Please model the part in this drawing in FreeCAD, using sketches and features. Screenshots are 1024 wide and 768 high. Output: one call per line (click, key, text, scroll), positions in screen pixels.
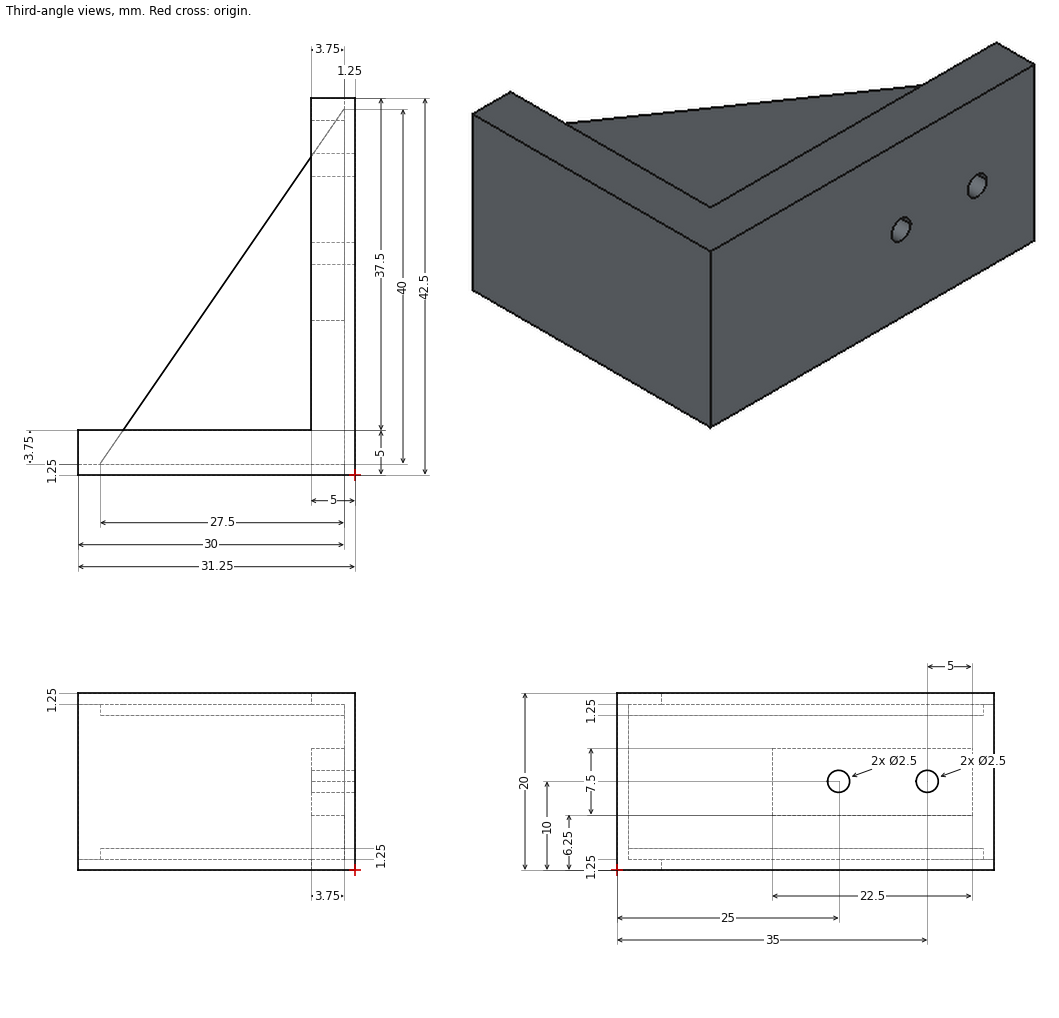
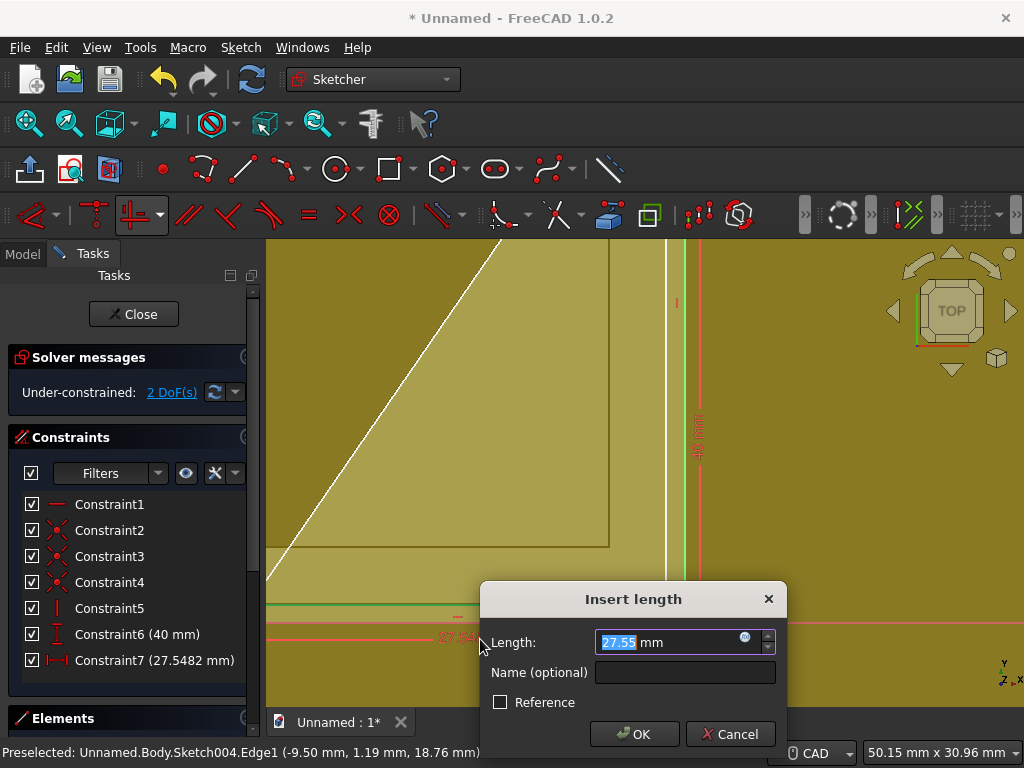
text(27.5)
key(Return)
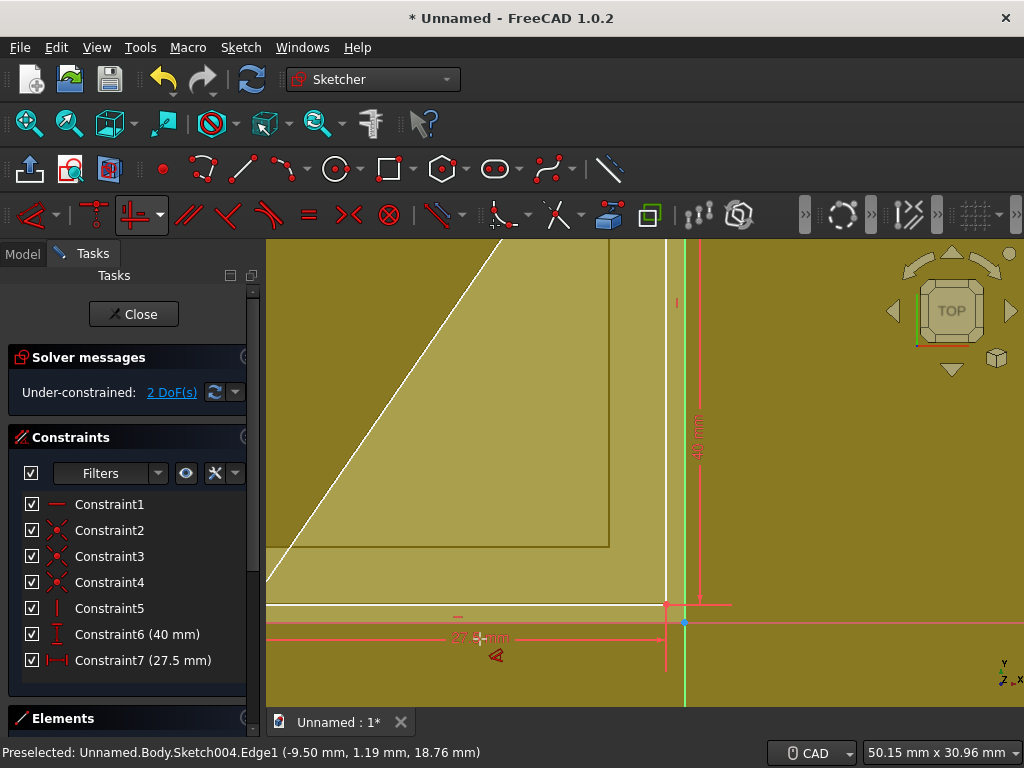
scroll(666, 605, up, 4)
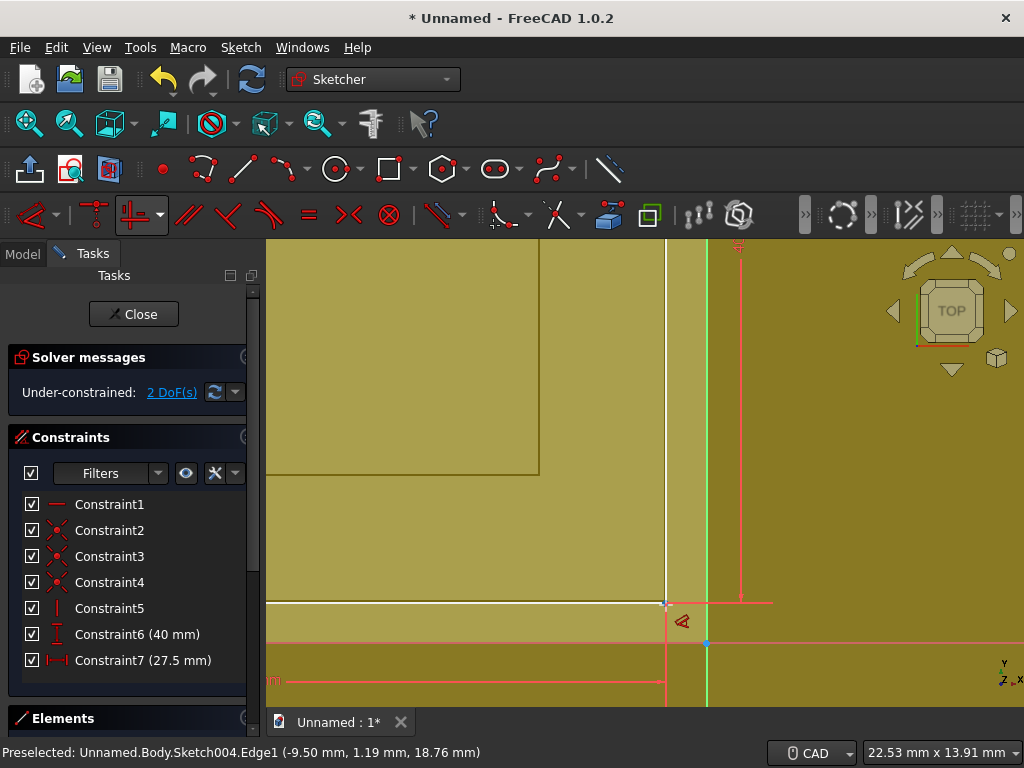
click(666, 603)
click(686, 677)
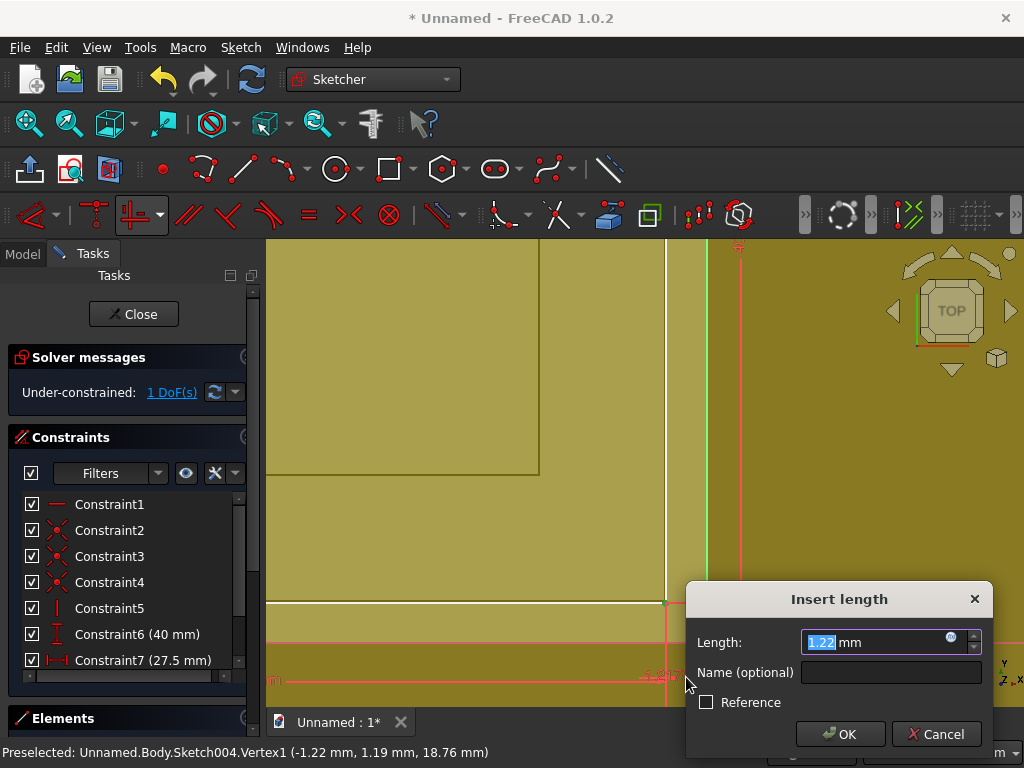
text(1.25)
key(Return)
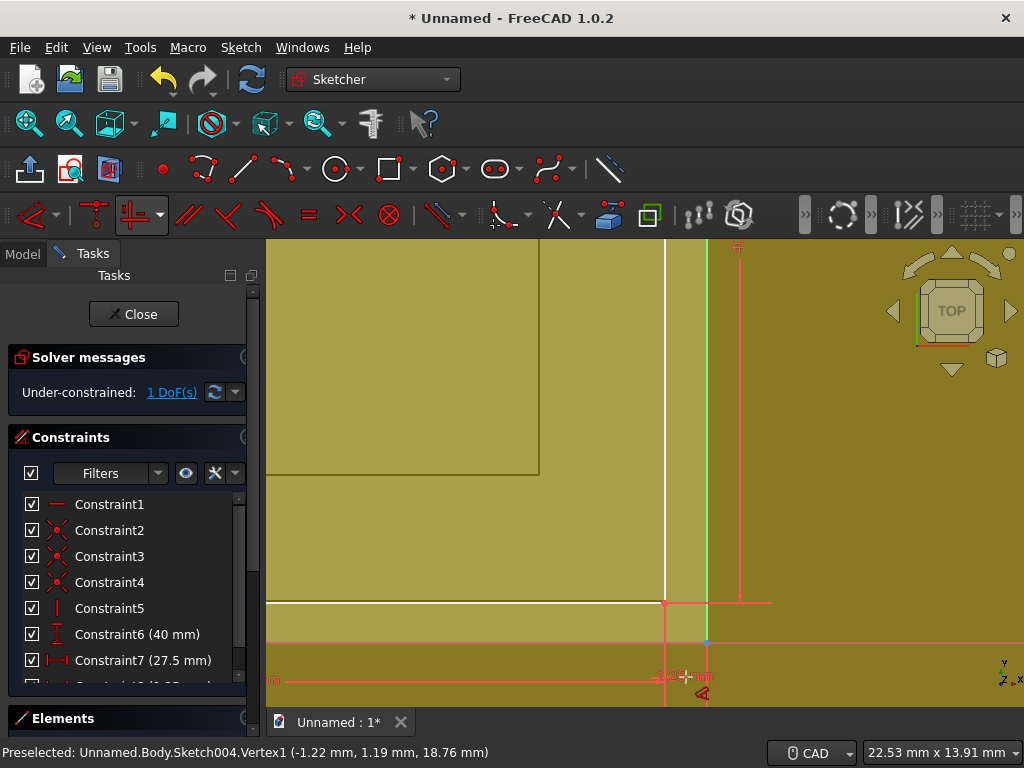
click(665, 603)
click(741, 623)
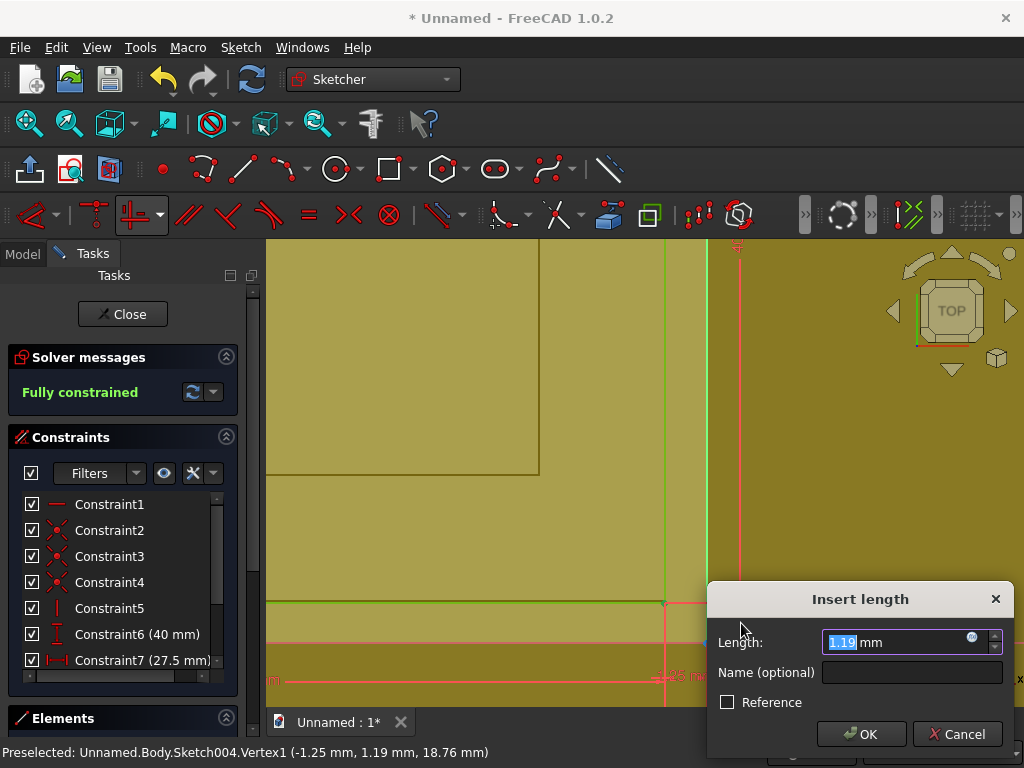
text(1.25)
key(Return)
key(Escape)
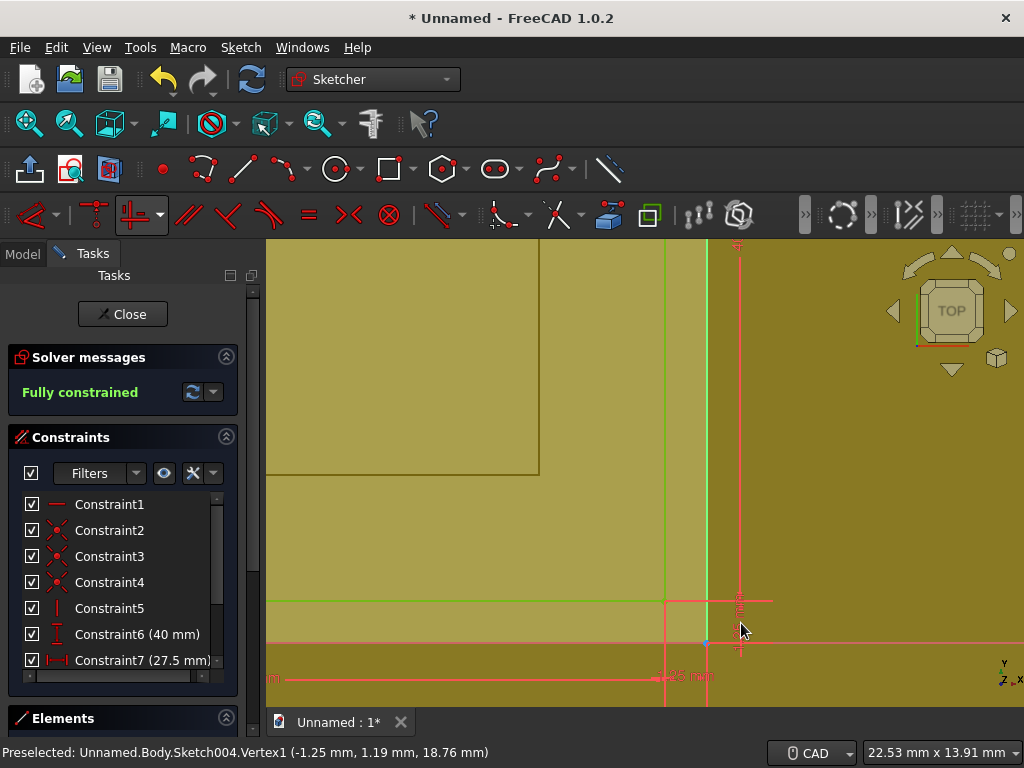
click(123, 314)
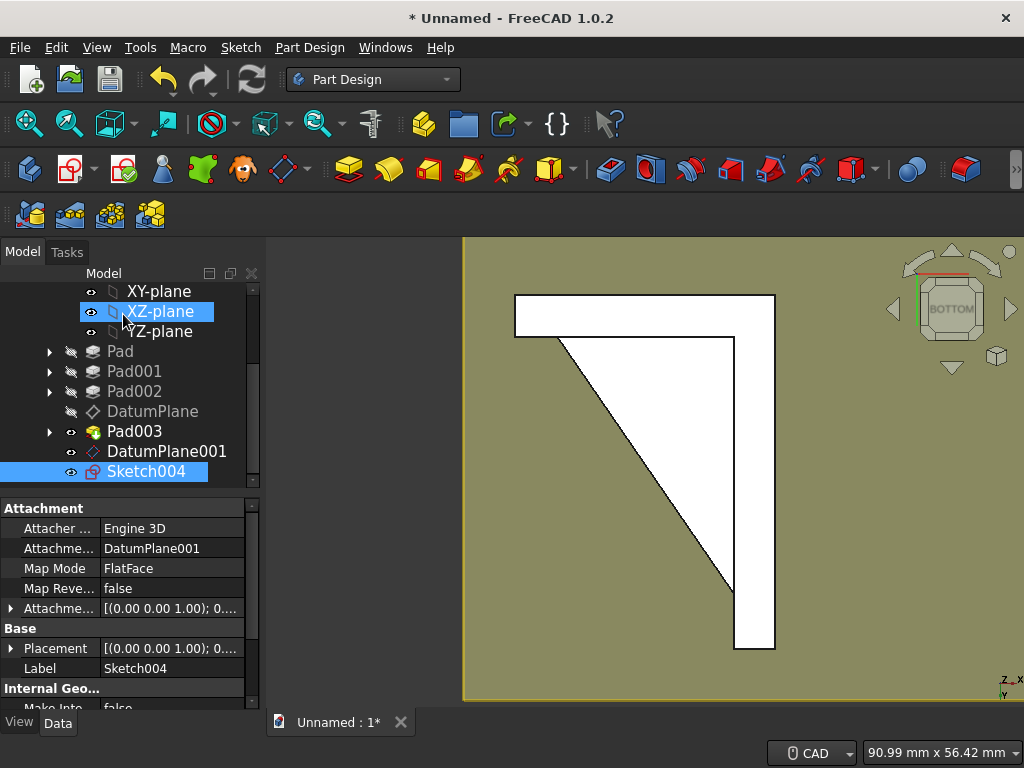
click(350, 170)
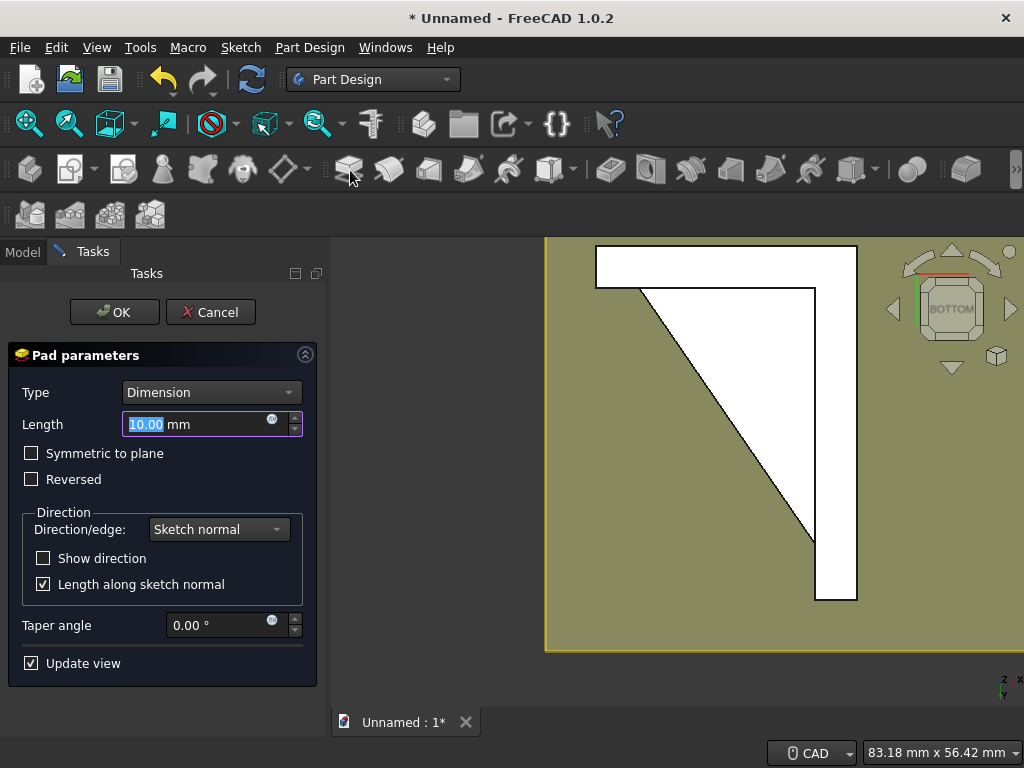
text(1.25)
key(Tab)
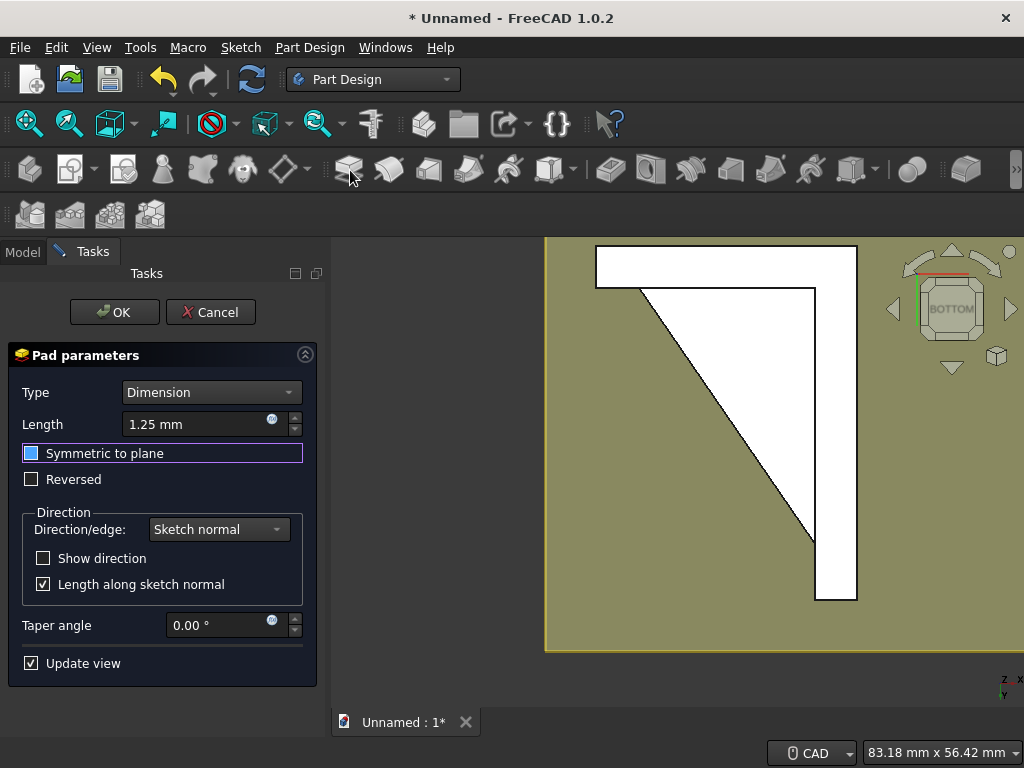
click(30, 479)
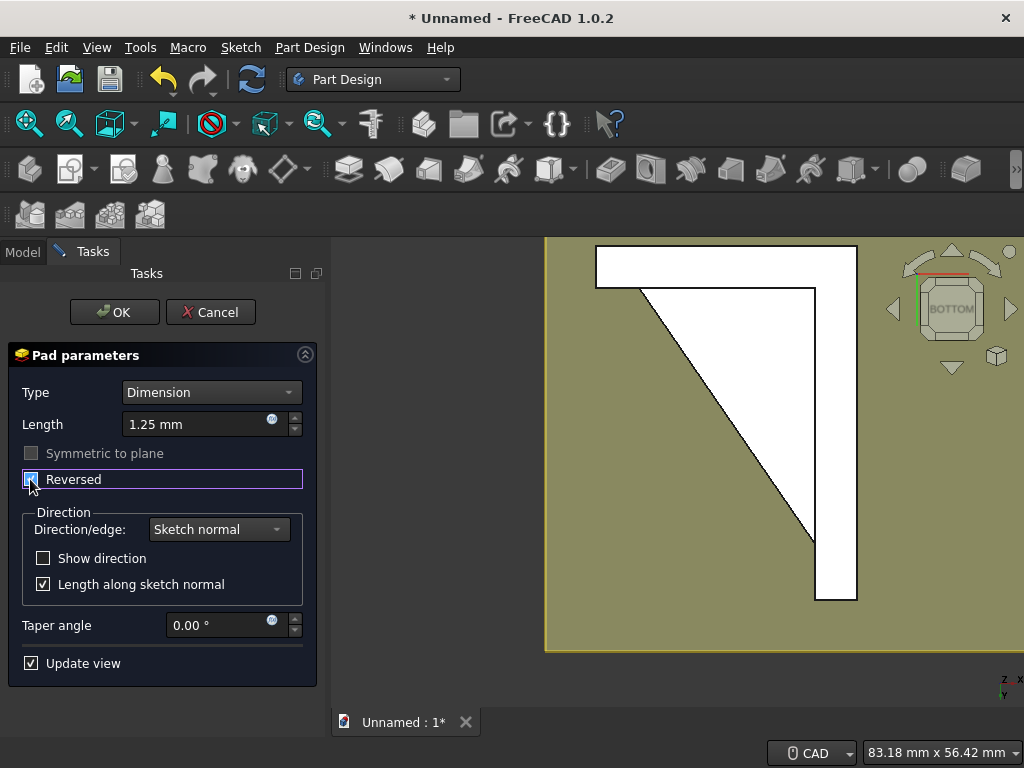
click(115, 312)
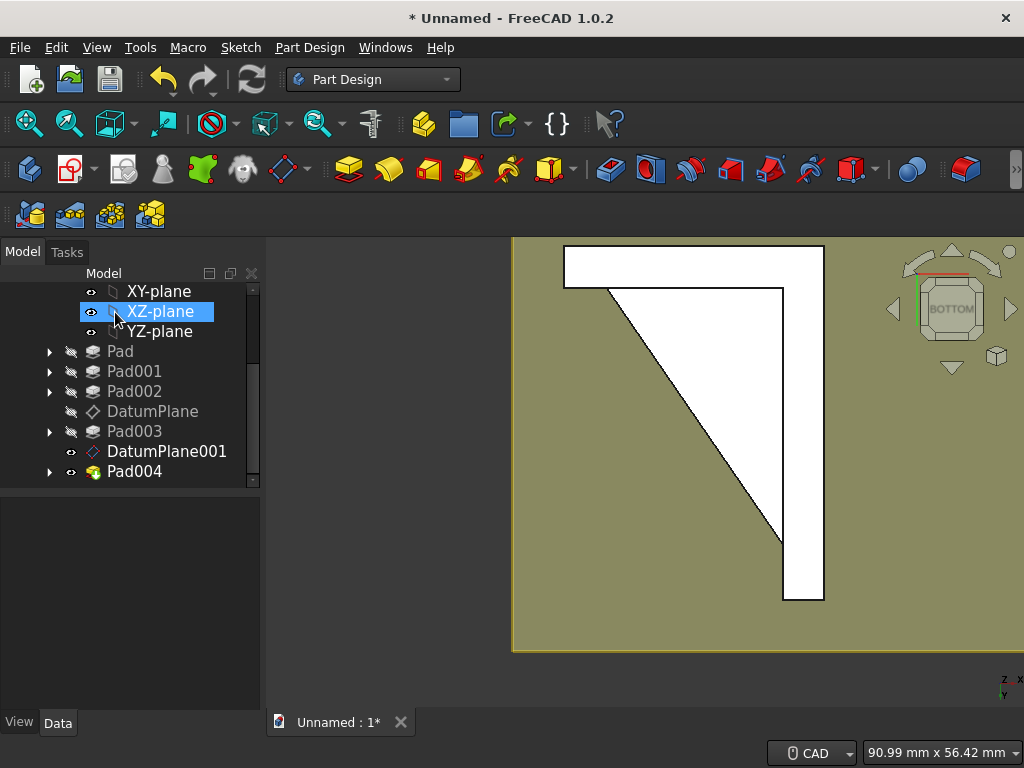
click(116, 452)
key(space)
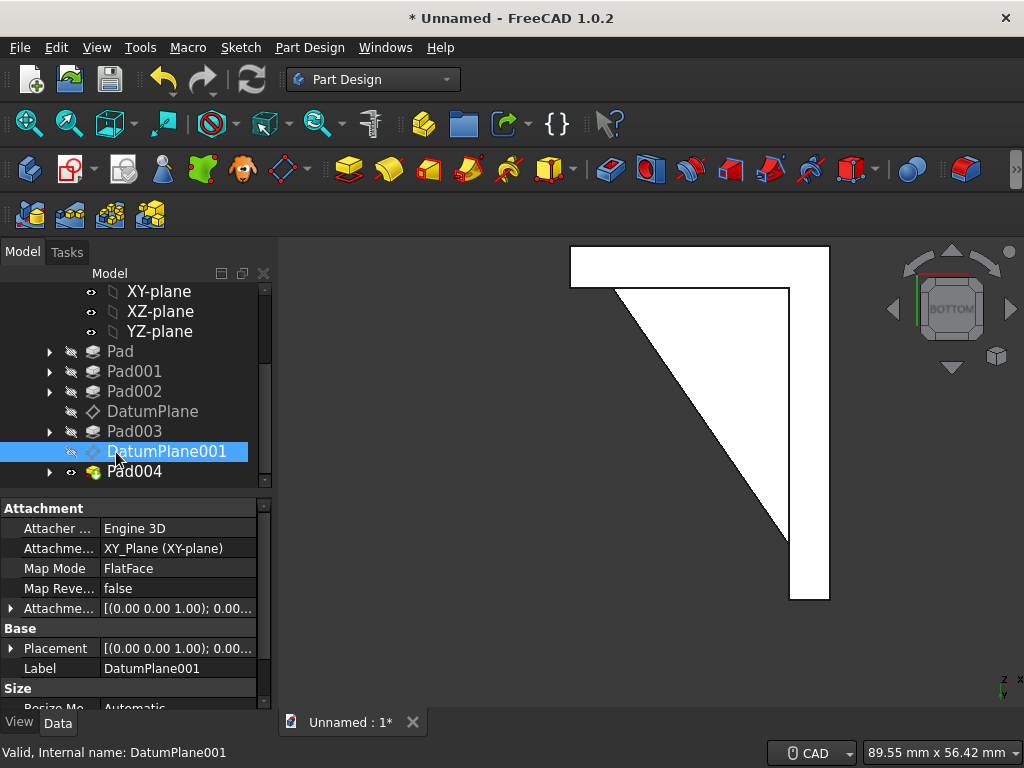
key(6)